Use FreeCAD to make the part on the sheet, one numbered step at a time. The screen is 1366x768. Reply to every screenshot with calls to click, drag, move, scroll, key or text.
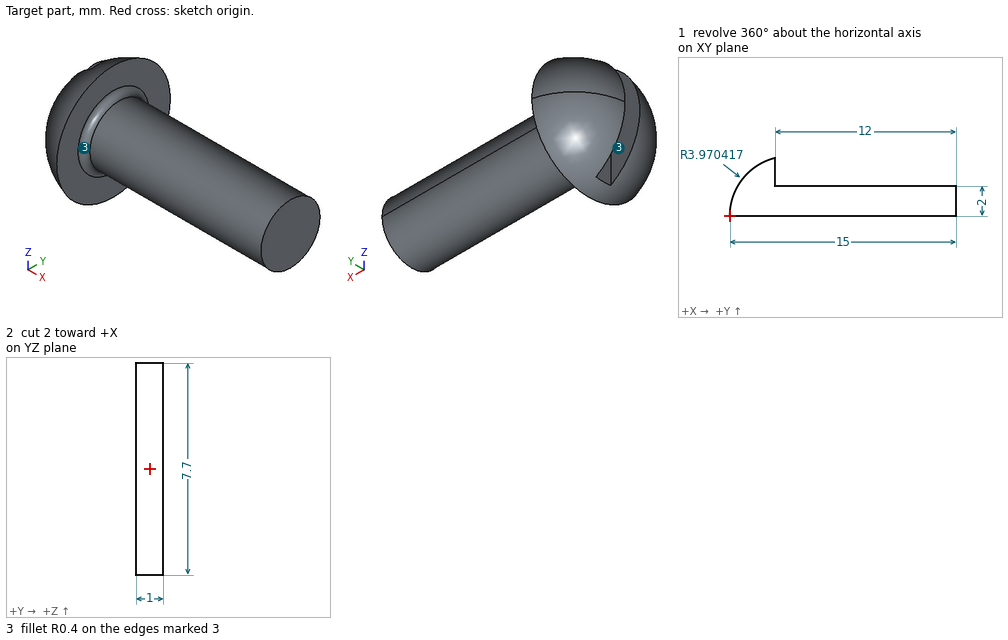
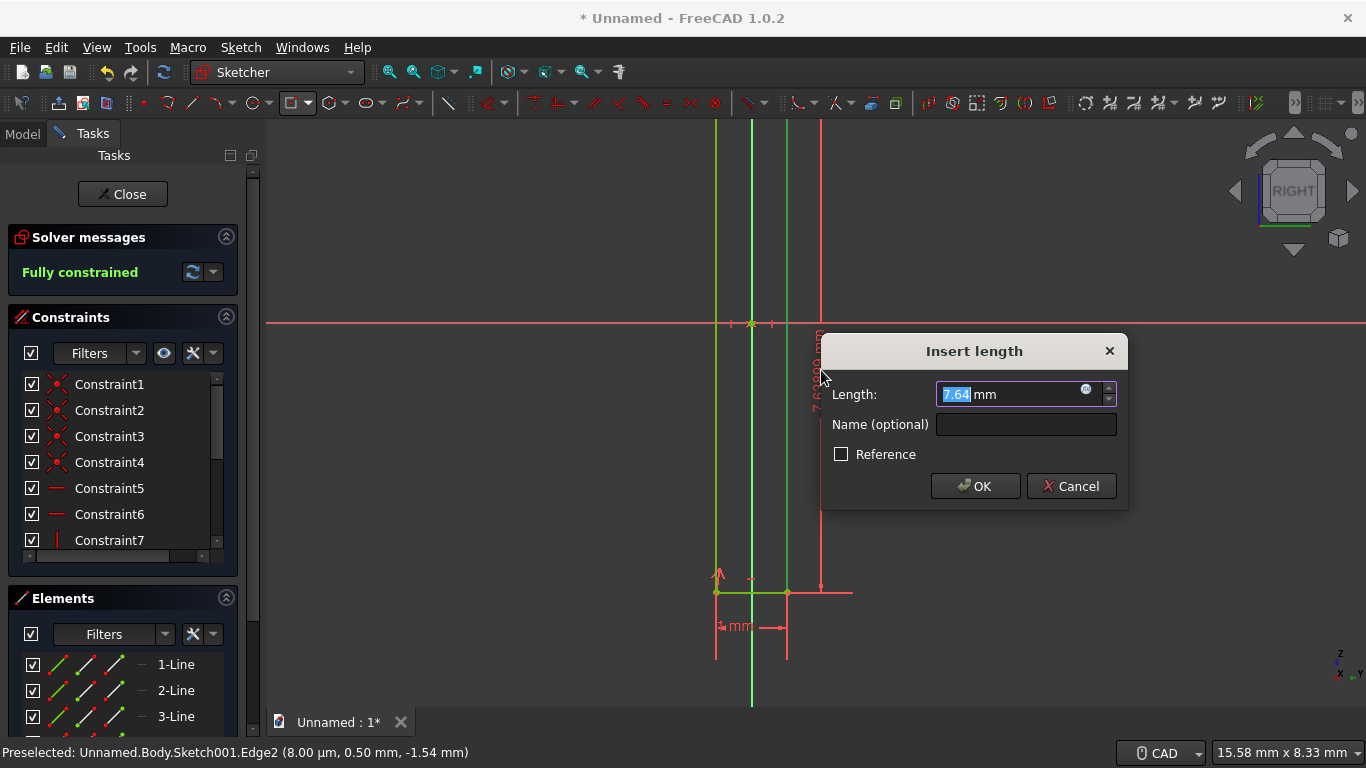
text(7.7)
key(Return)
key(Escape)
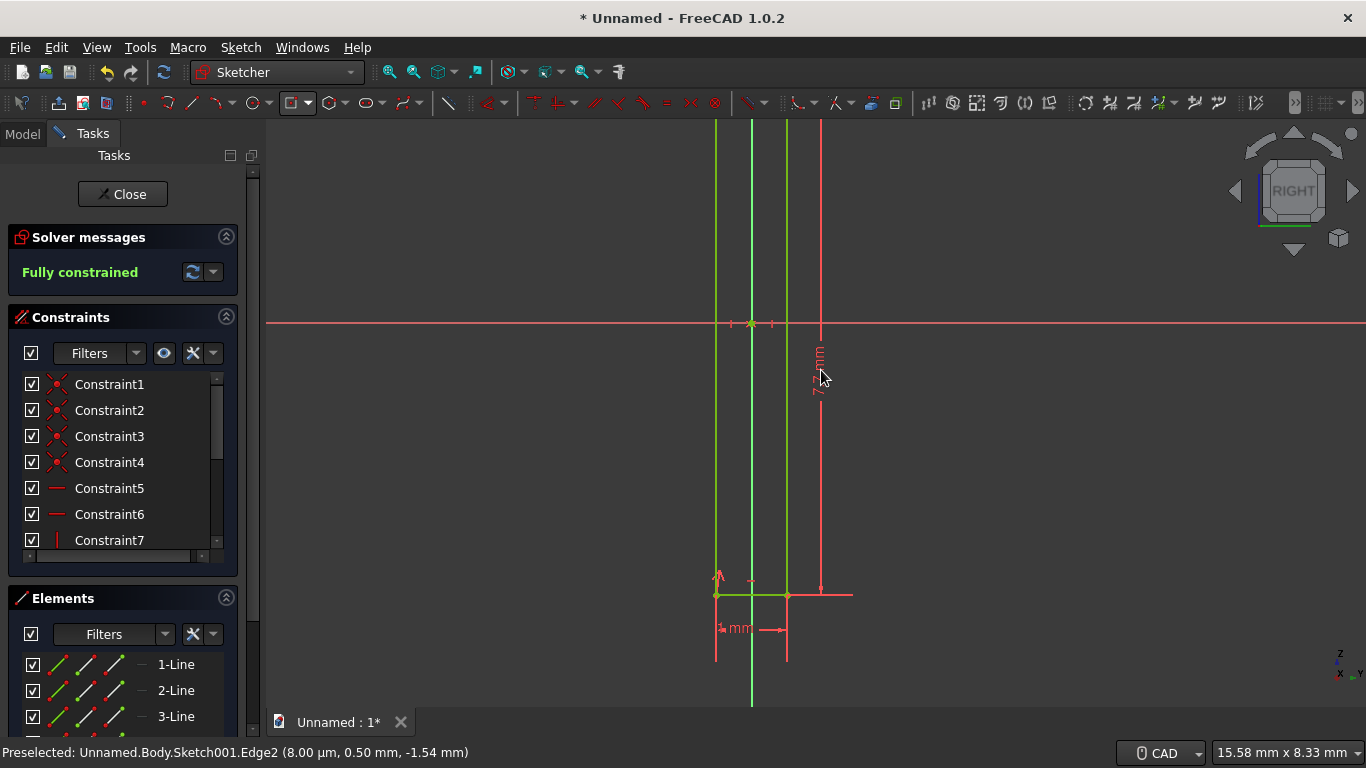
click(123, 194)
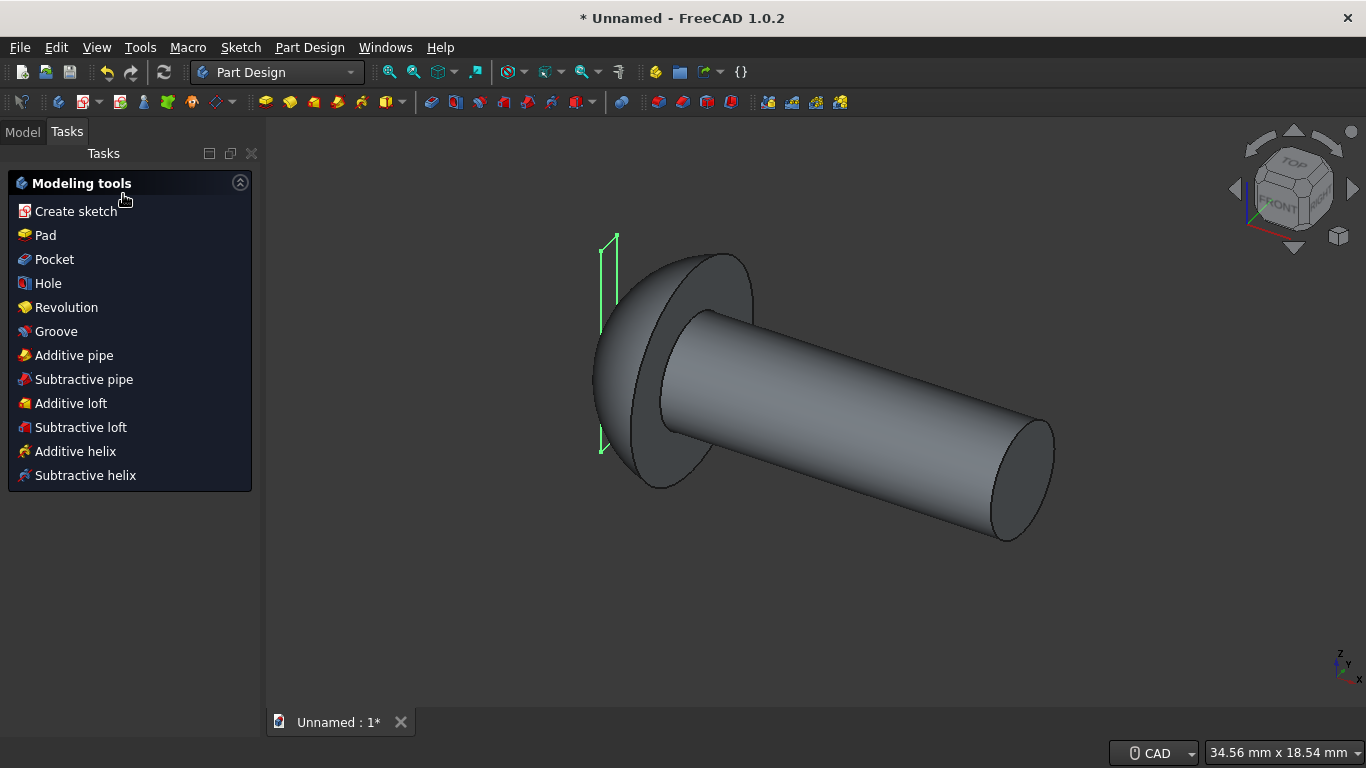
click(432, 102)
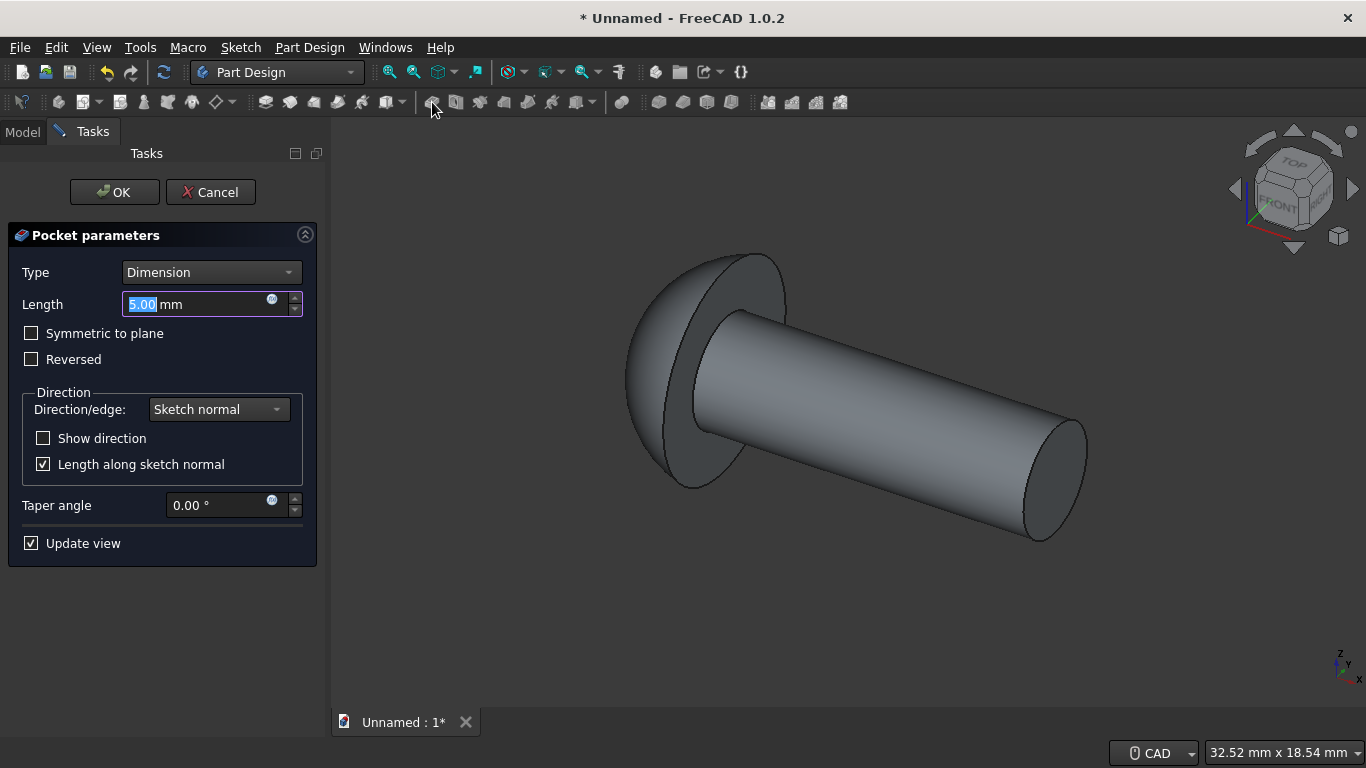
text(2)
key(Tab)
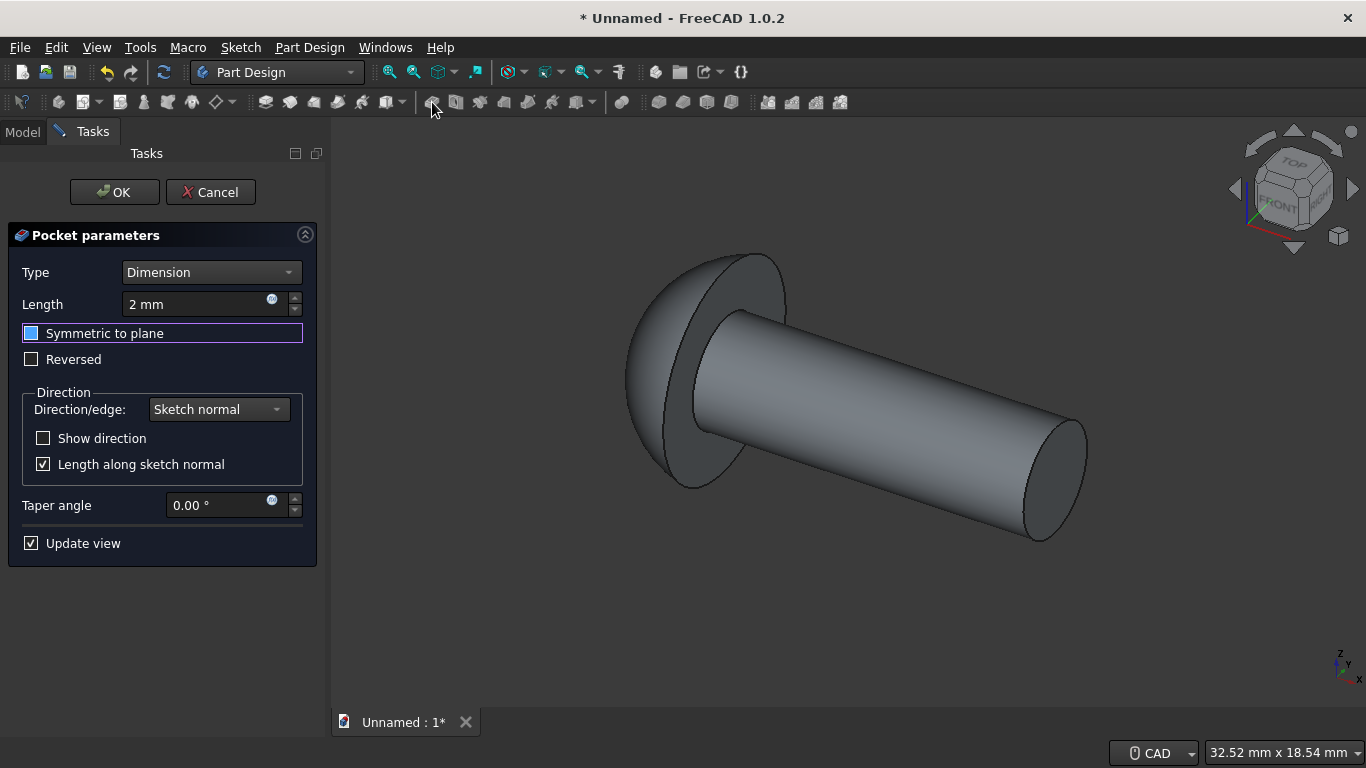
click(30, 359)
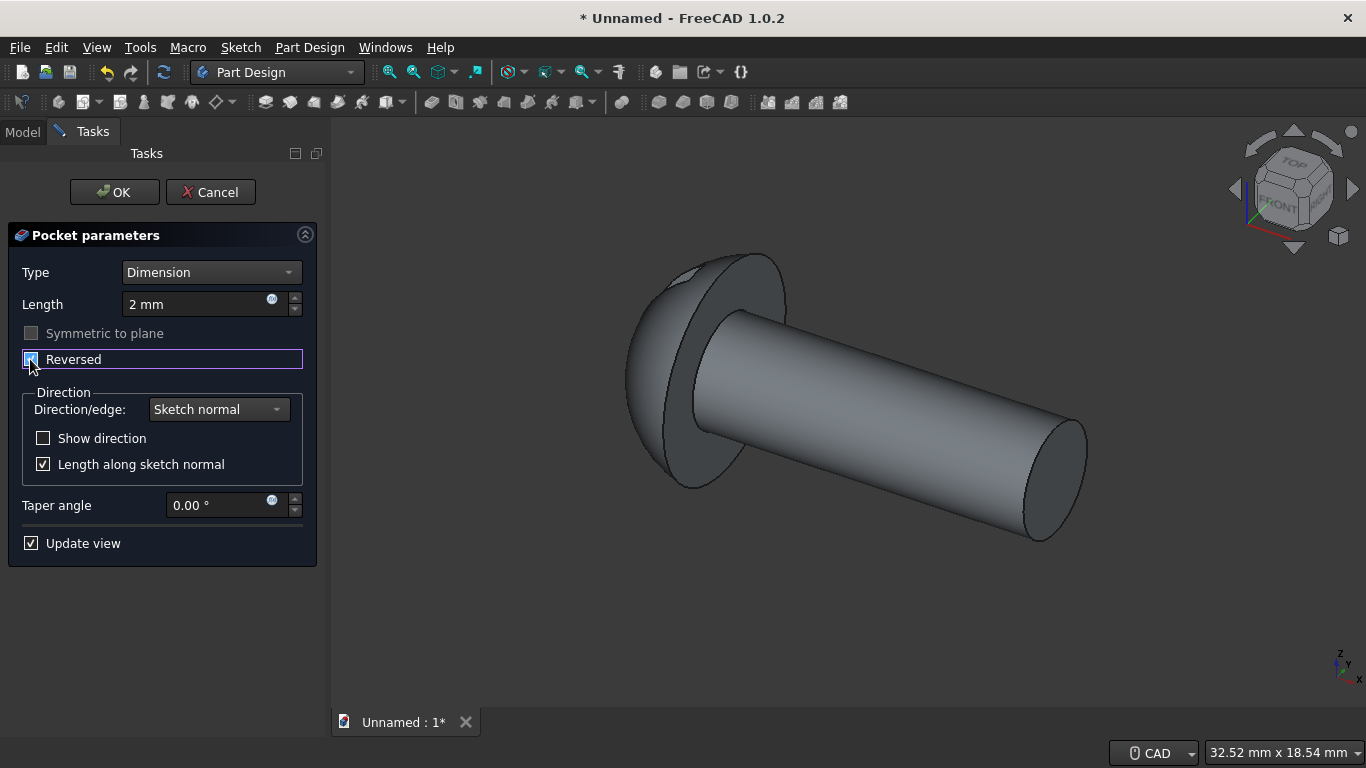
click(115, 192)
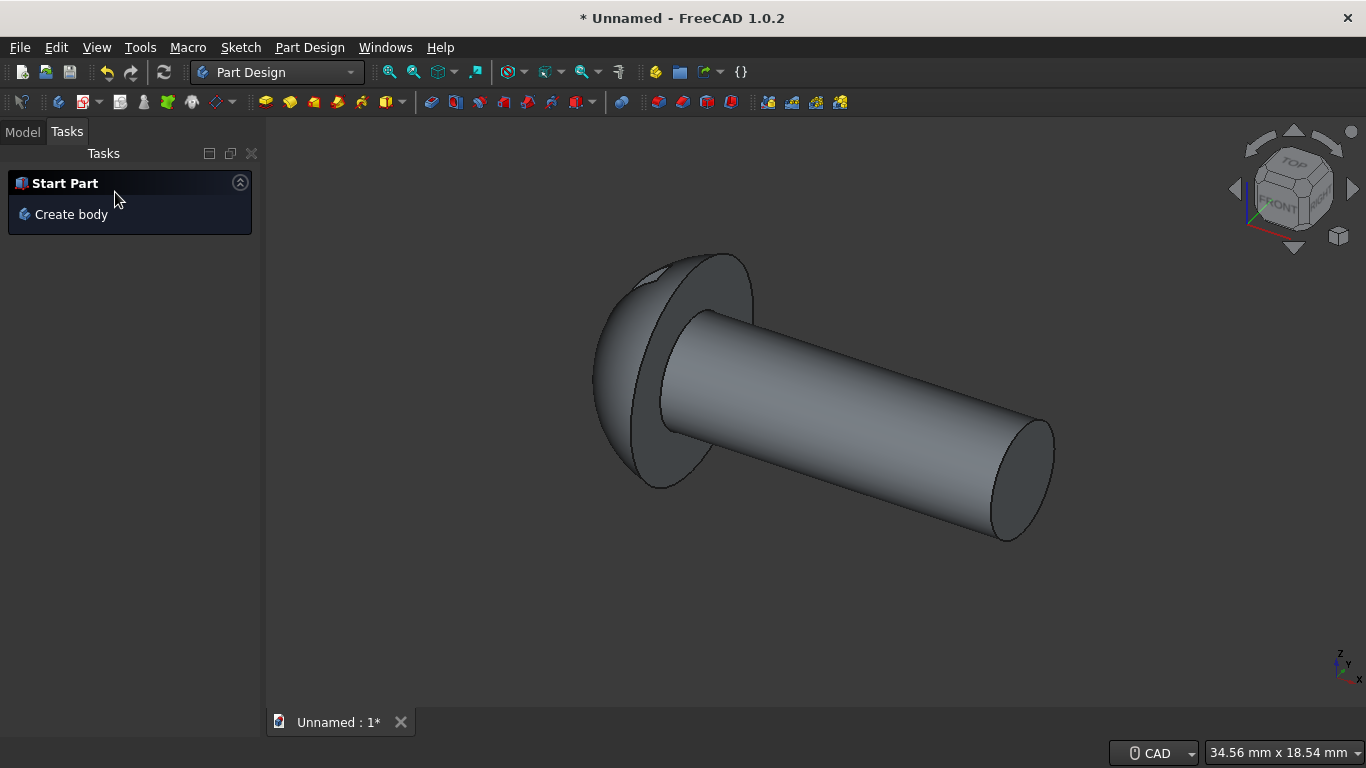
key(0)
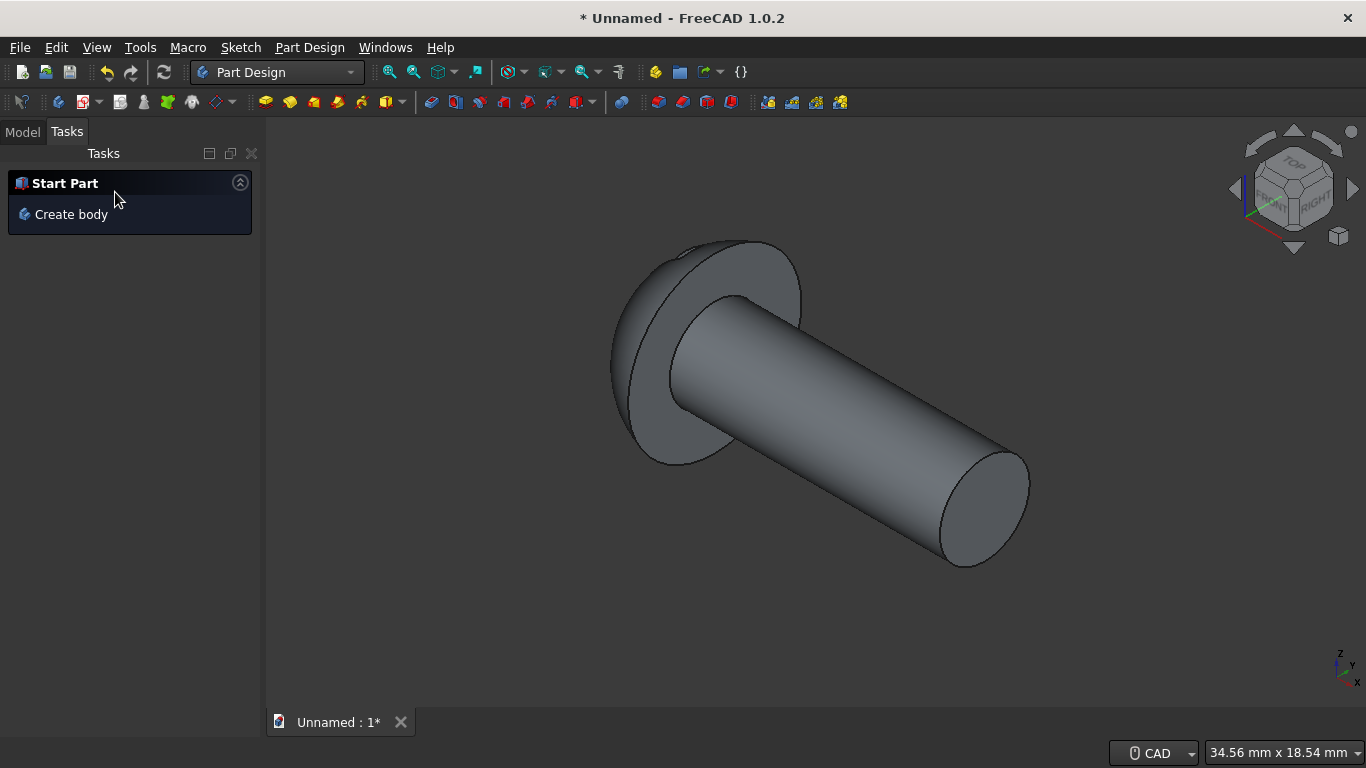
key(2)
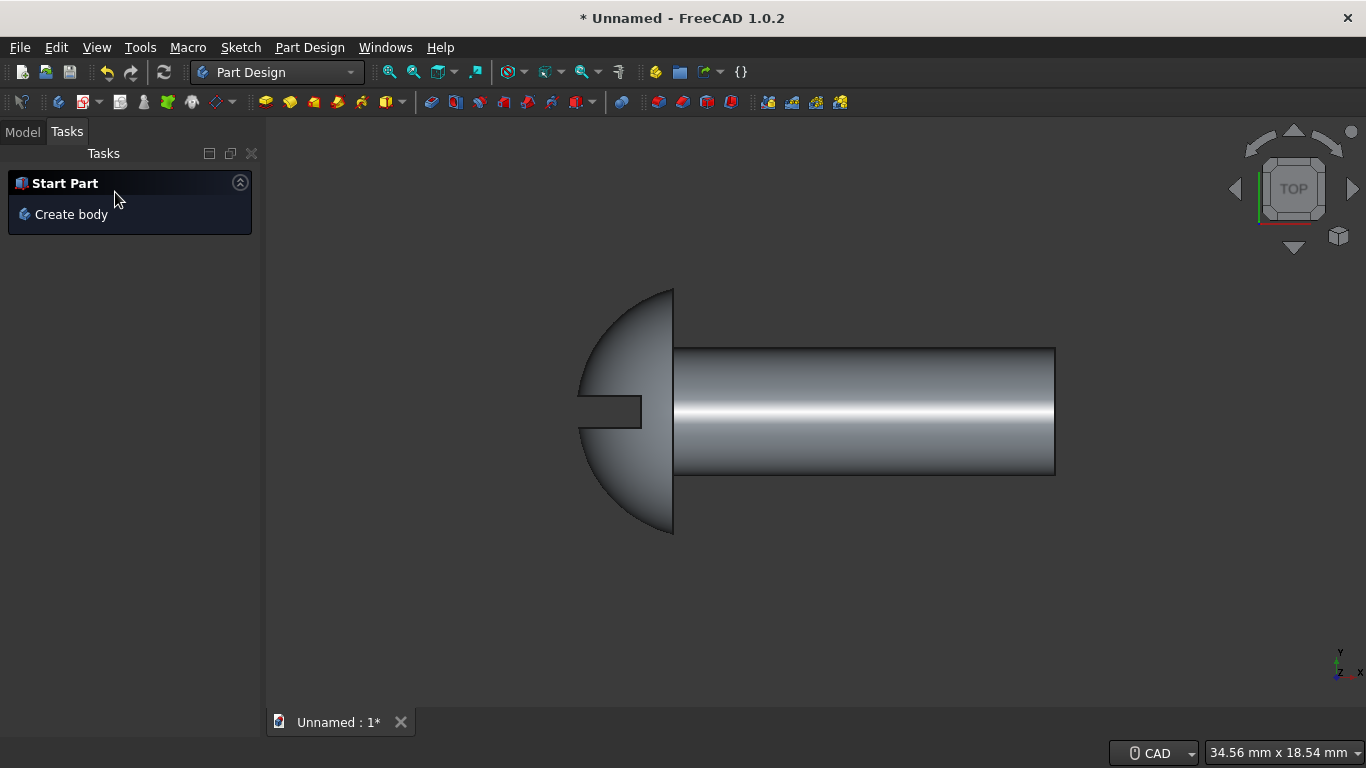
click(390, 72)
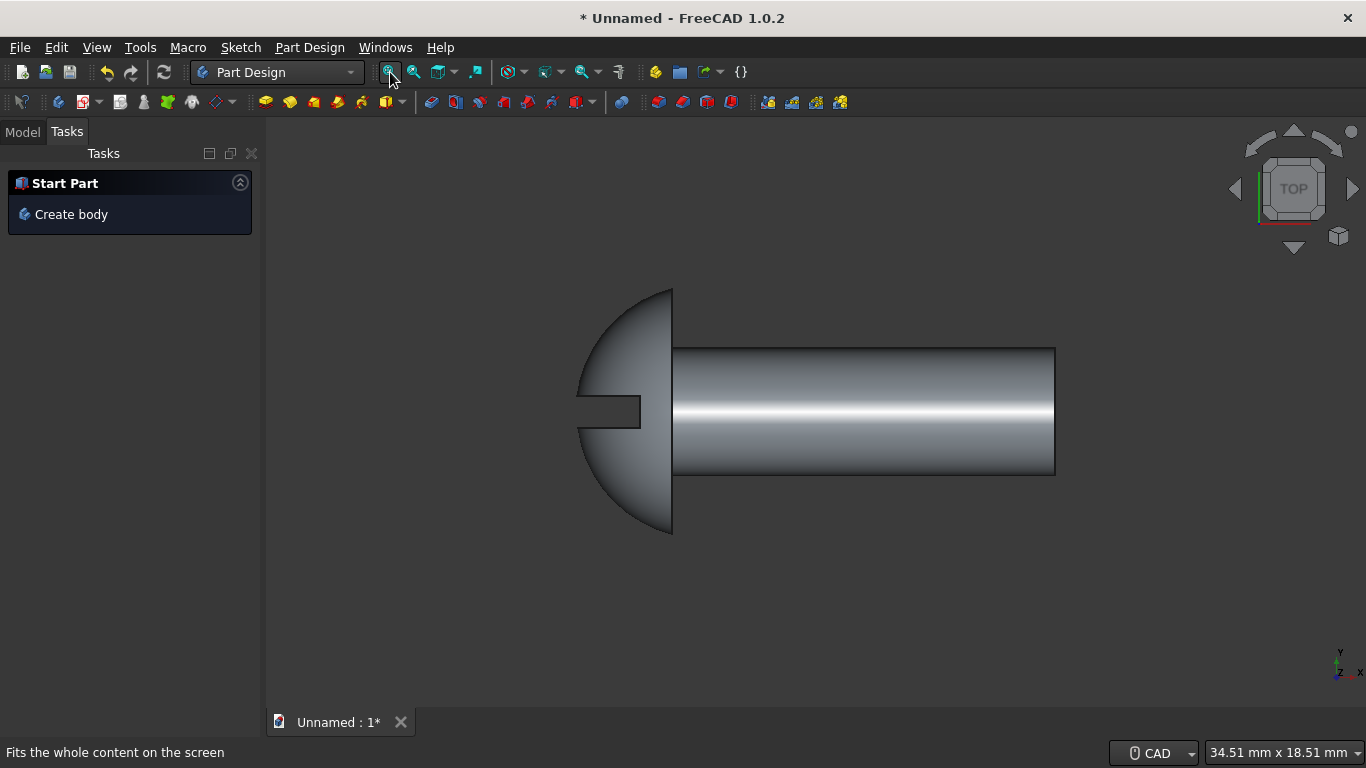
key(1)